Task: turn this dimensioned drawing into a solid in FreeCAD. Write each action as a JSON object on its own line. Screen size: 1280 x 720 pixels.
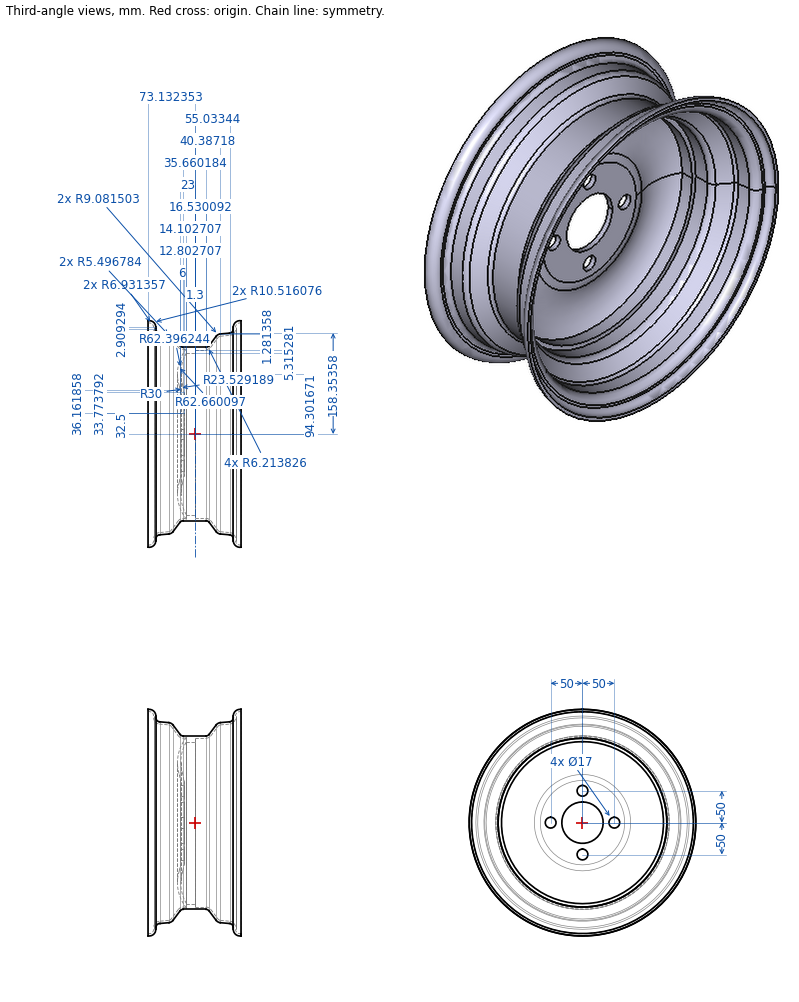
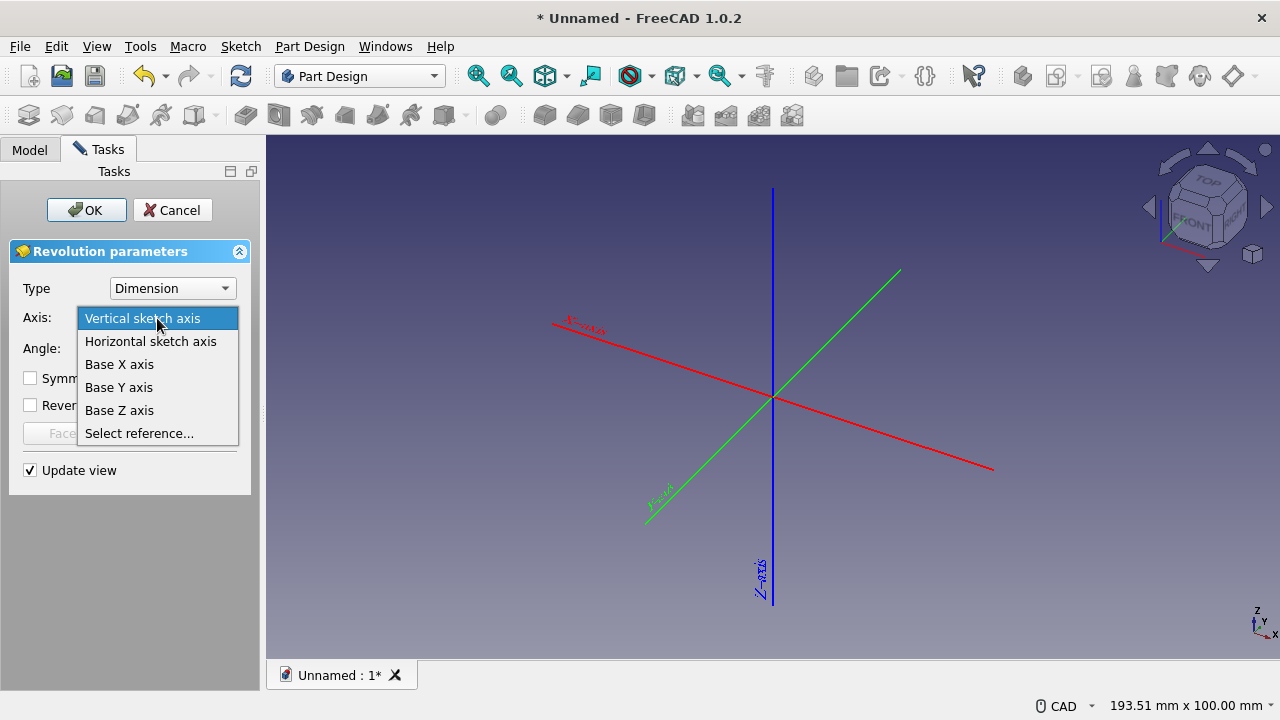
{"action": "left_click", "coordinate": [156, 342]}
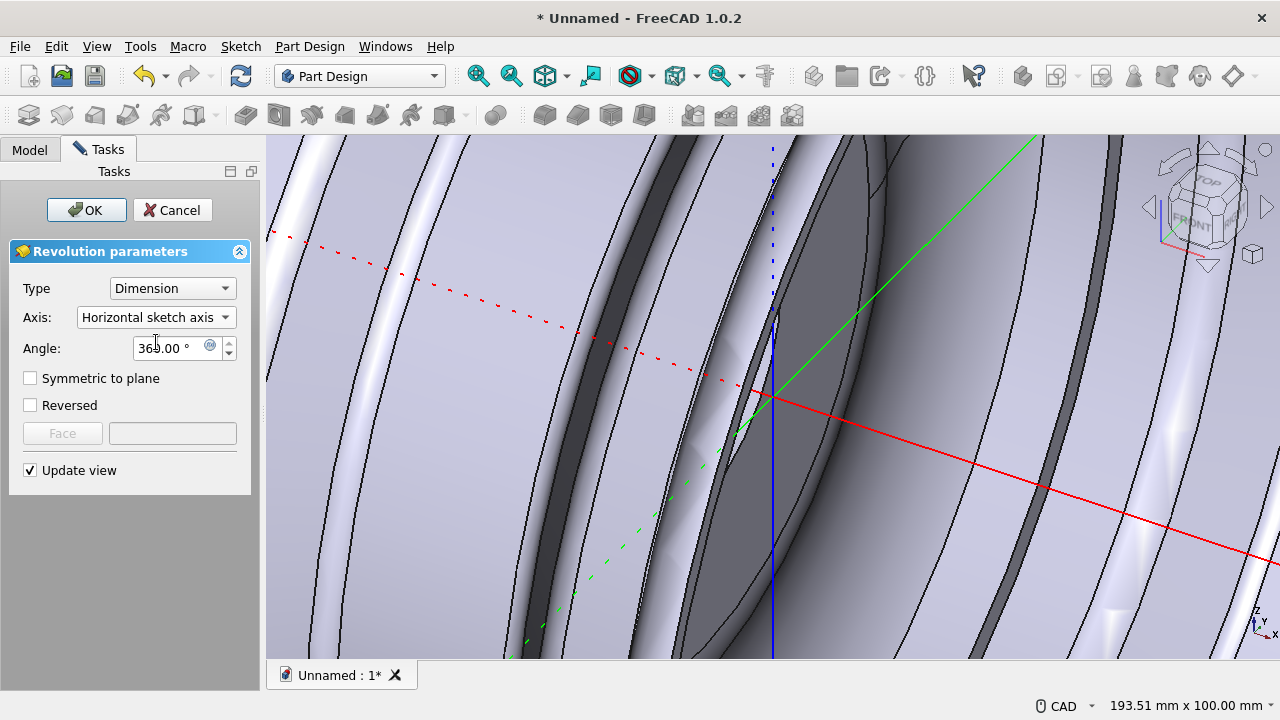
{"action": "left_click", "coordinate": [87, 210]}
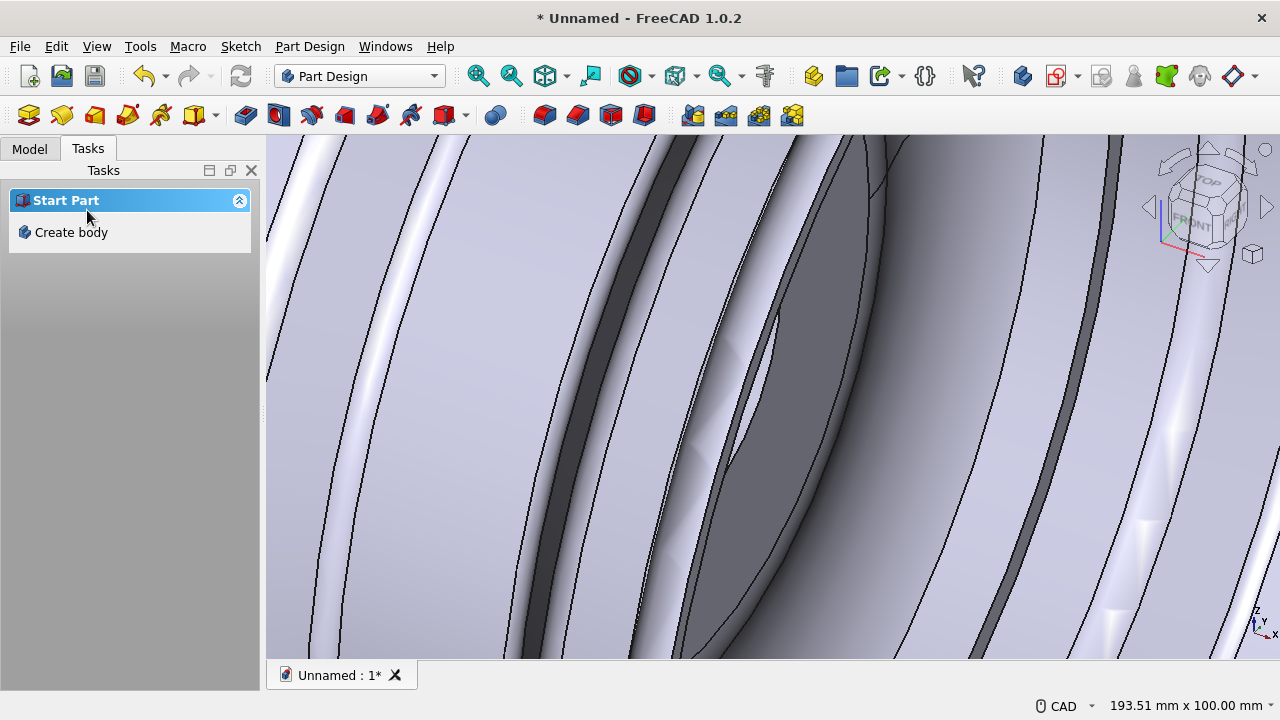
{"action": "left_click", "coordinate": [479, 76]}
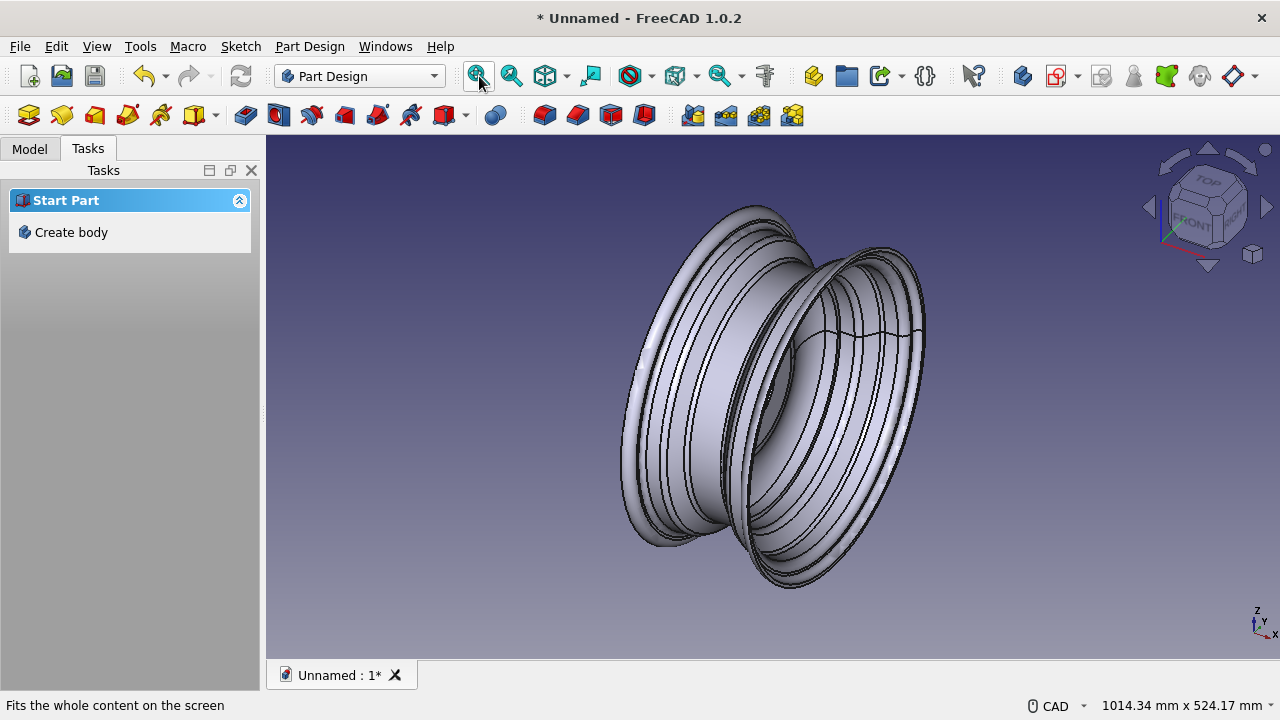
{"action": "key", "text": "6"}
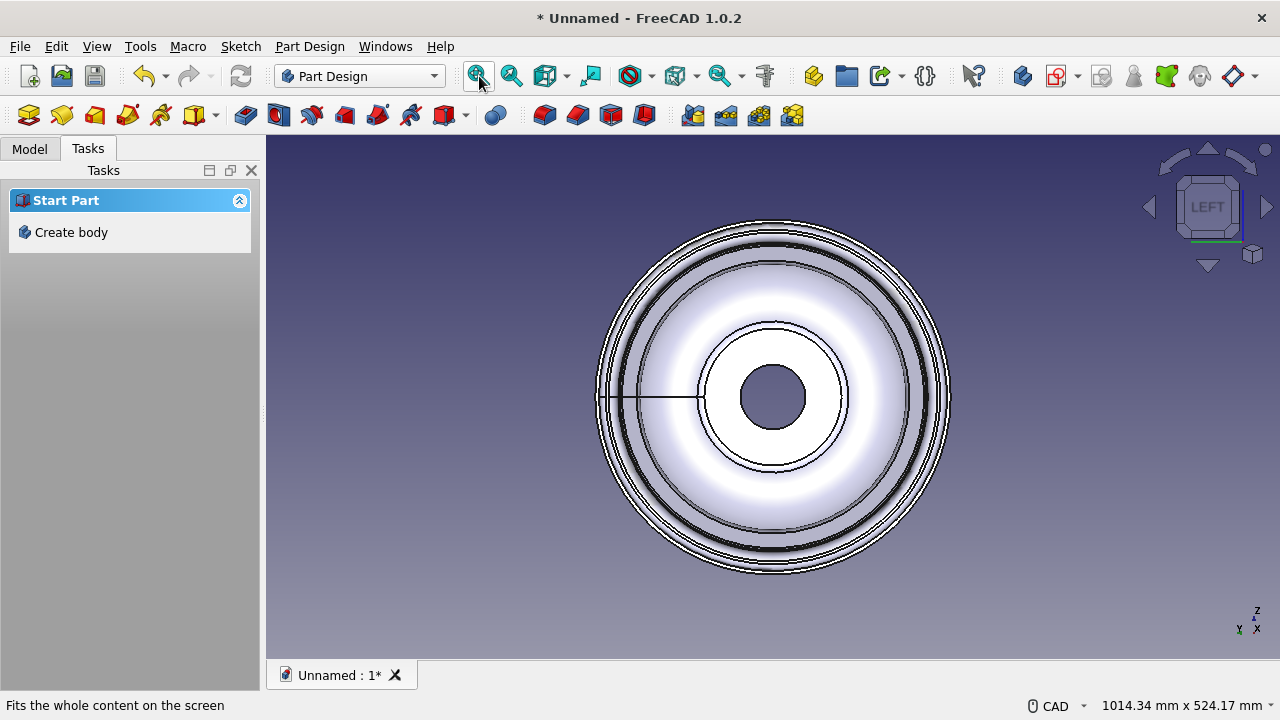
{"action": "left_click", "coordinate": [812, 435]}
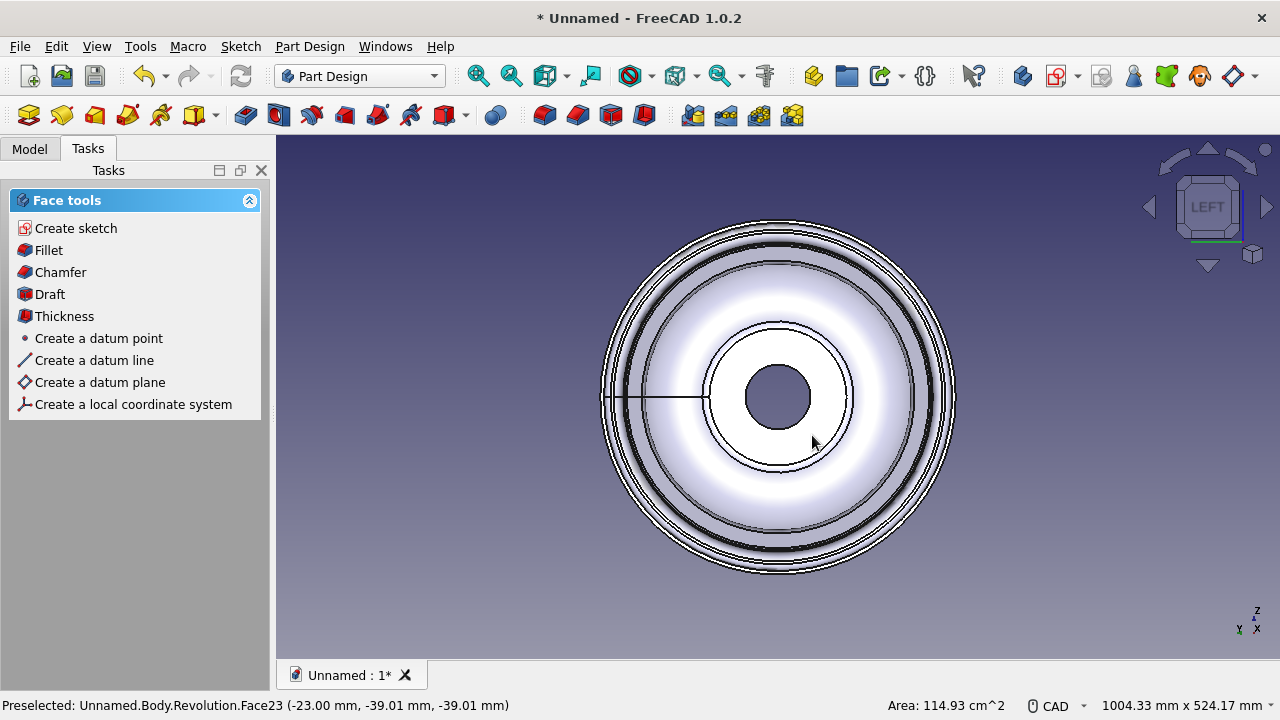
{"action": "left_click", "coordinate": [1056, 76]}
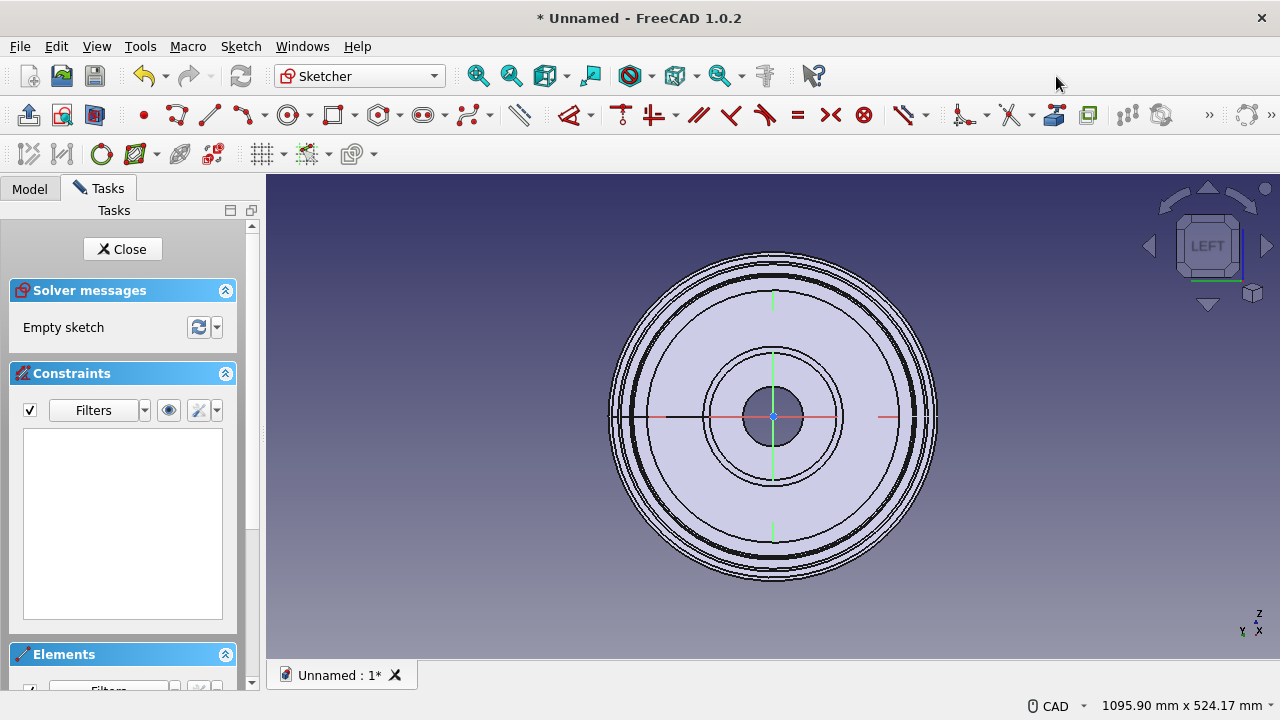
{"action": "key", "text": "q s"}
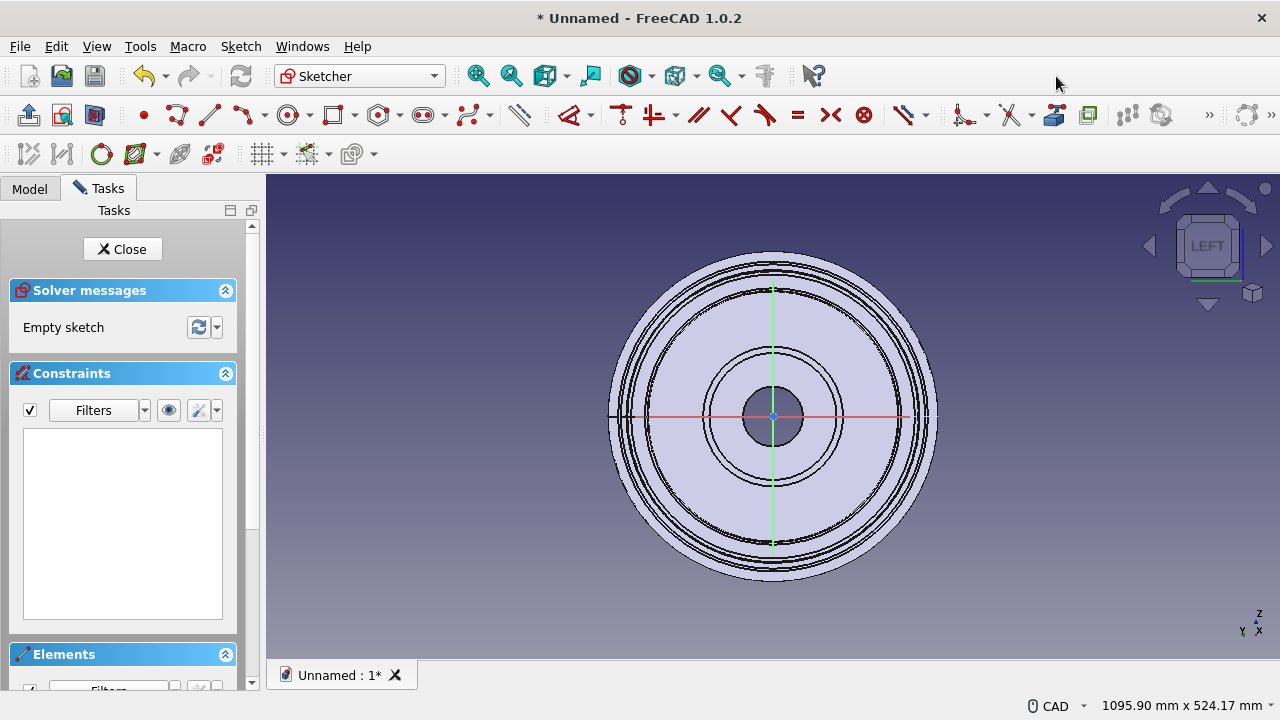
{"action": "scroll", "coordinate": [813, 416], "scroll_direction": "up", "scroll_amount": 5}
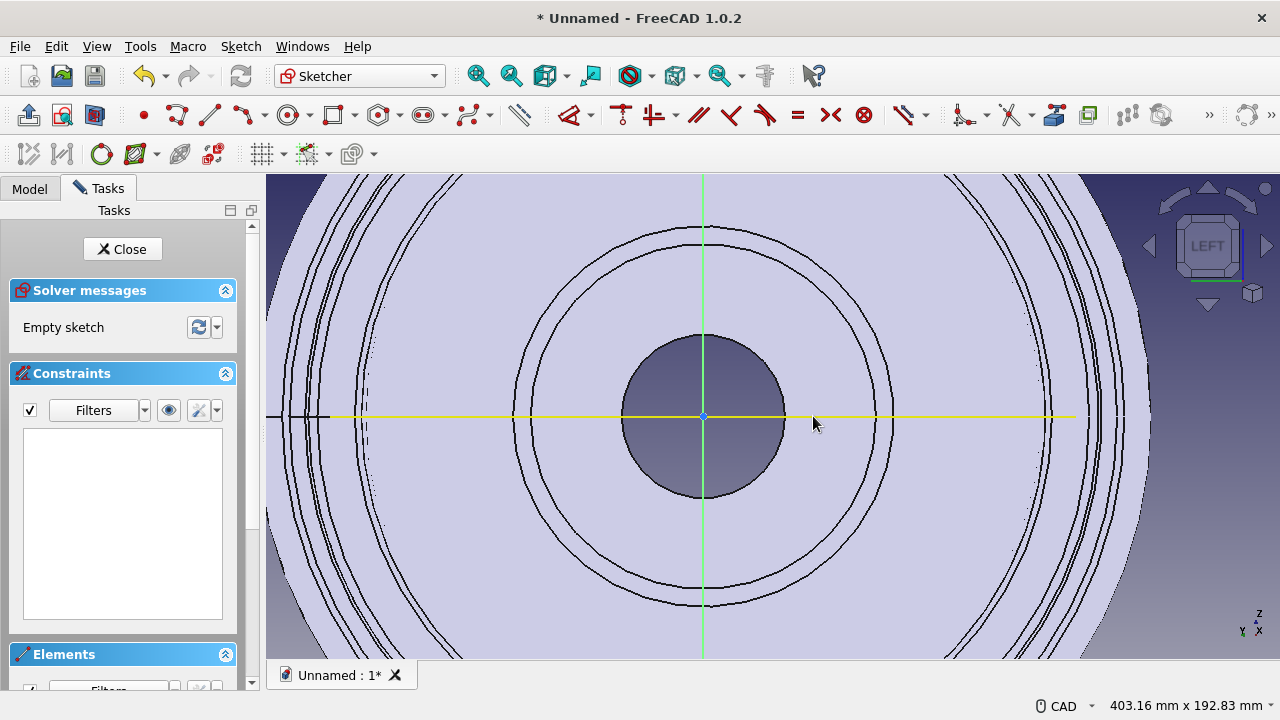
{"action": "left_click", "coordinate": [288, 116]}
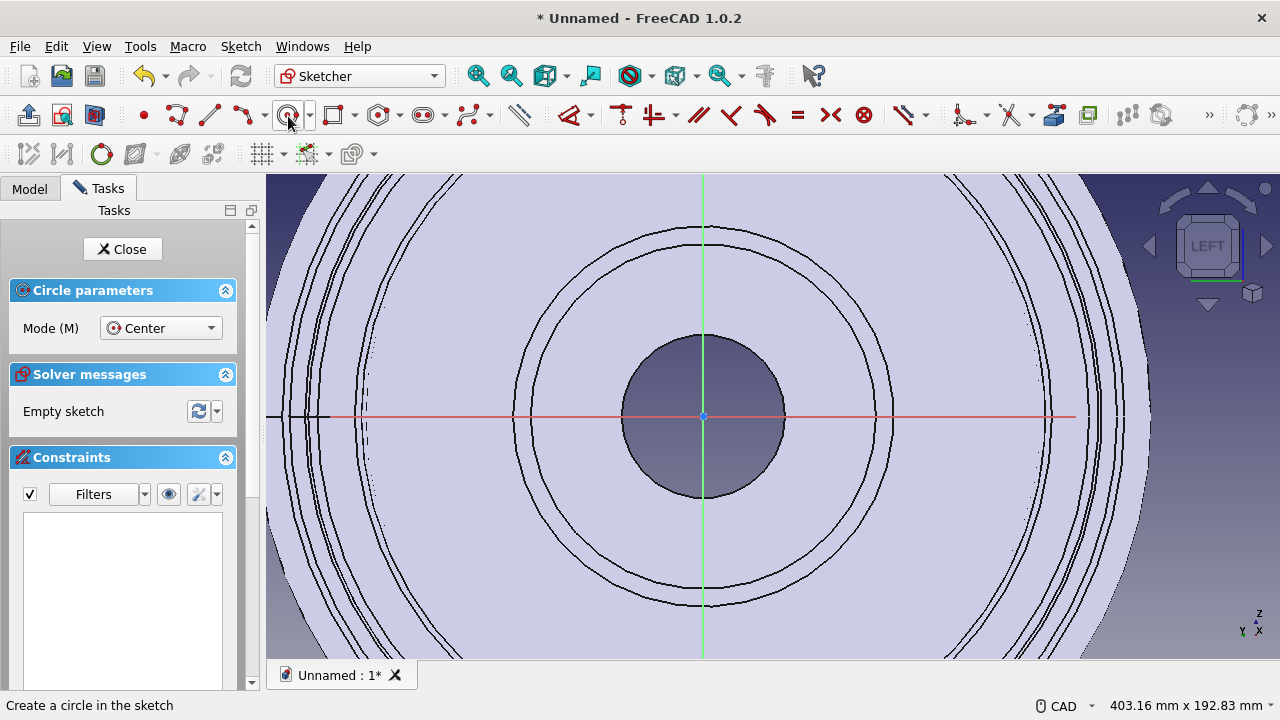
{"action": "left_click", "coordinate": [578, 416]}
{"action": "mouse_move", "coordinate": [593, 401]}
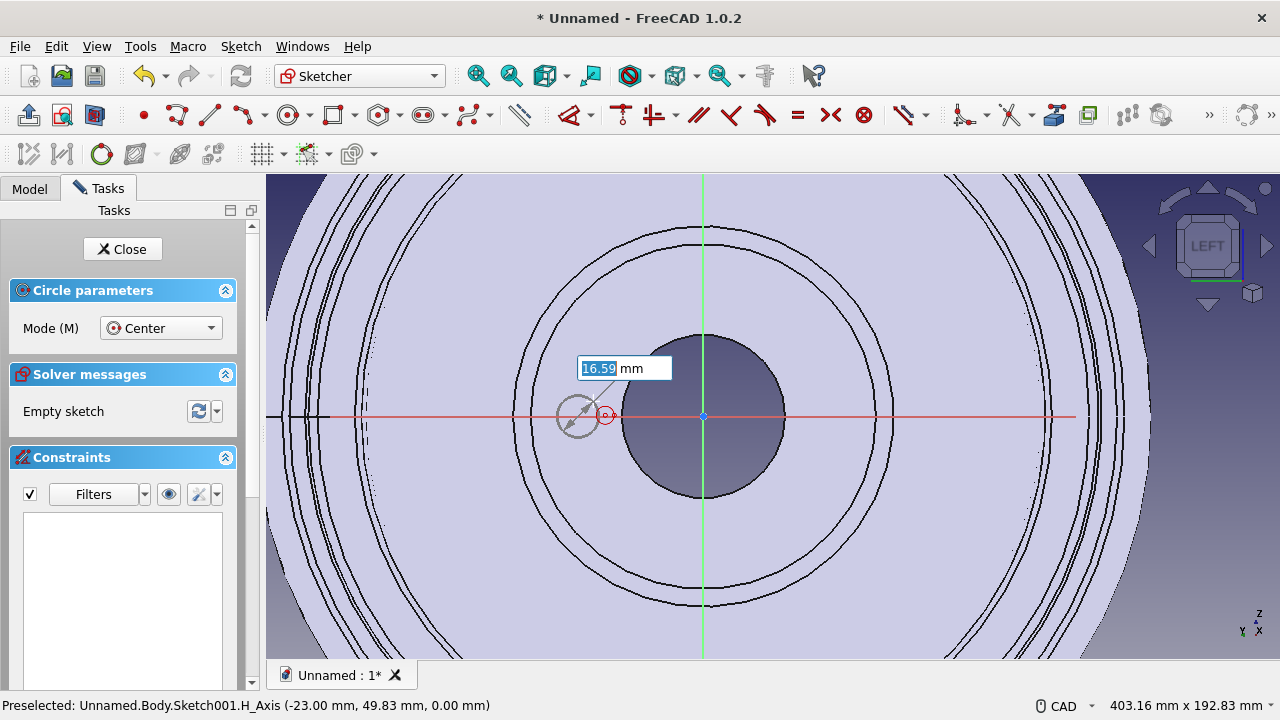
{"action": "type", "text": "17"}
{"action": "key", "text": "Return"}